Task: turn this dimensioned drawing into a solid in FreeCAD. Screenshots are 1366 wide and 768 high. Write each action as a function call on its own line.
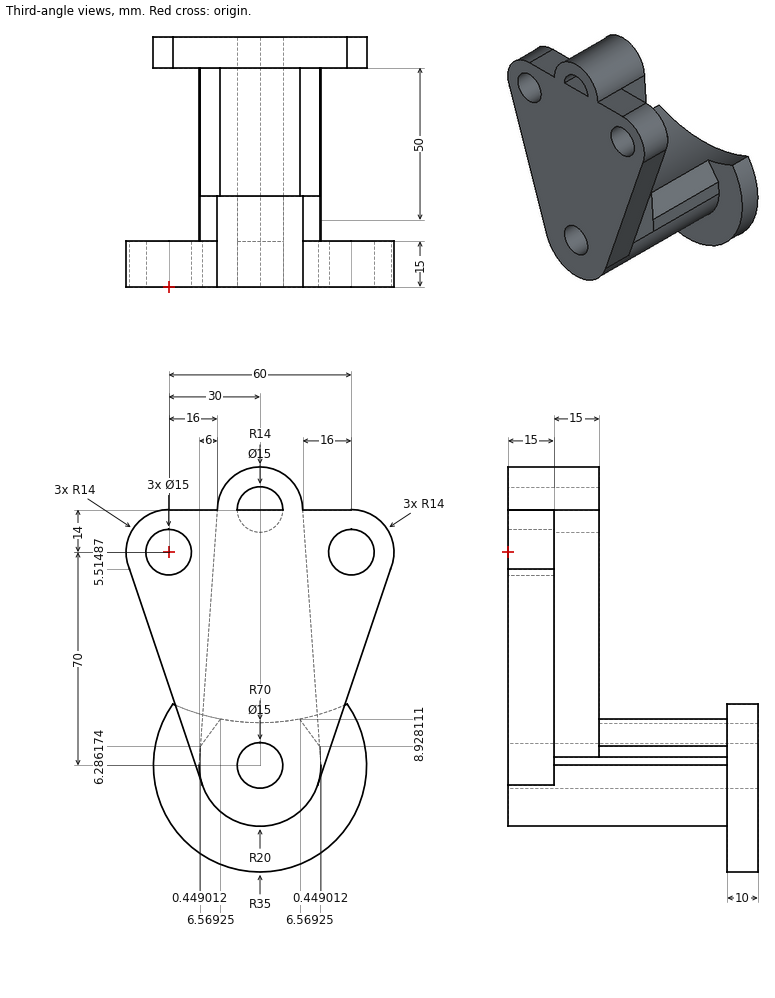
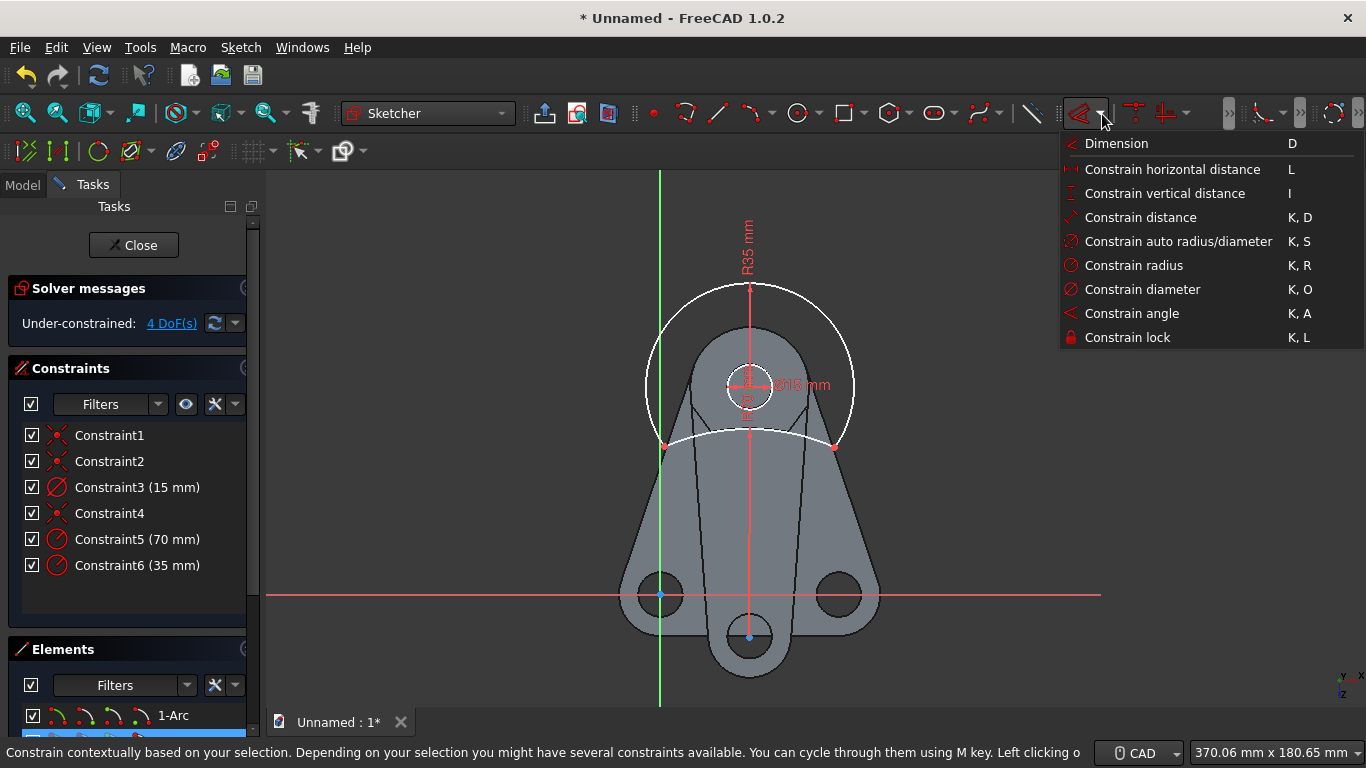
click(1212, 169)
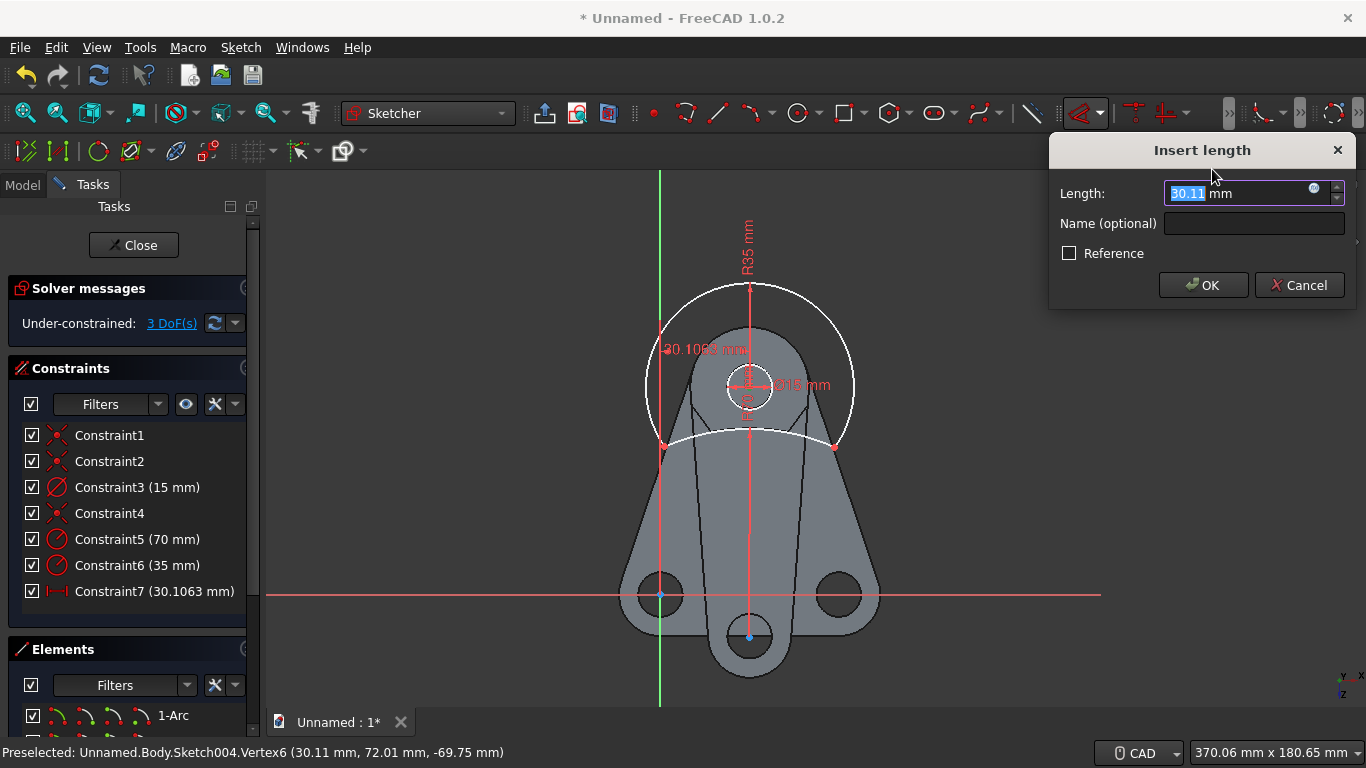
text(30)
key(Return)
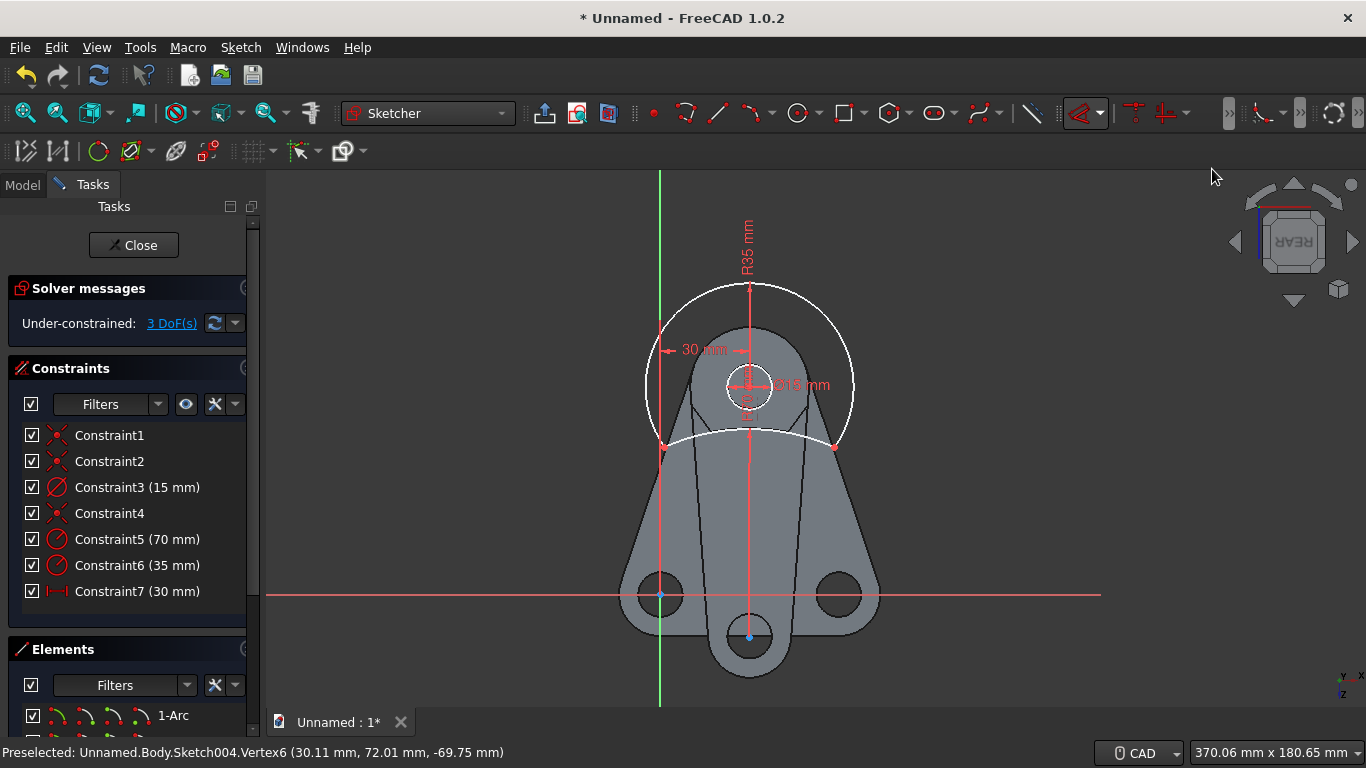
click(750, 387)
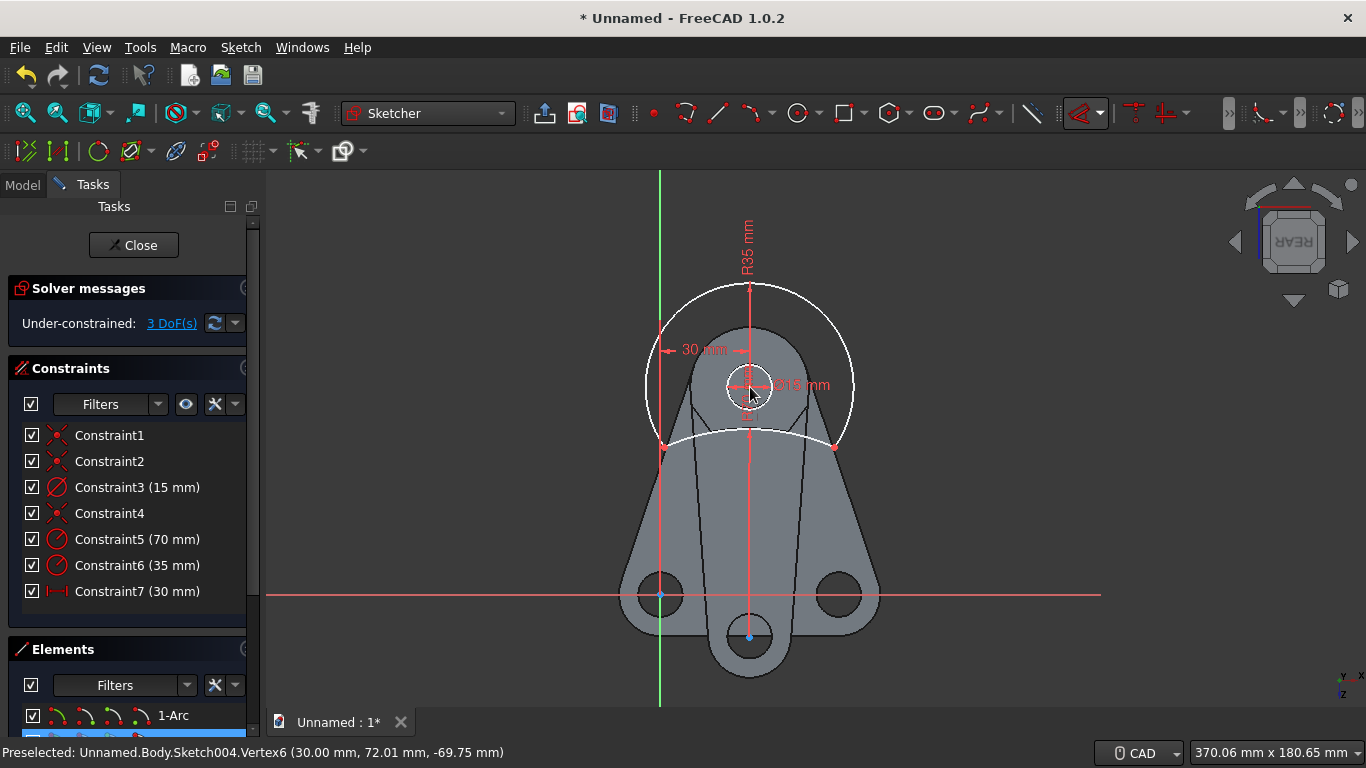
key(i)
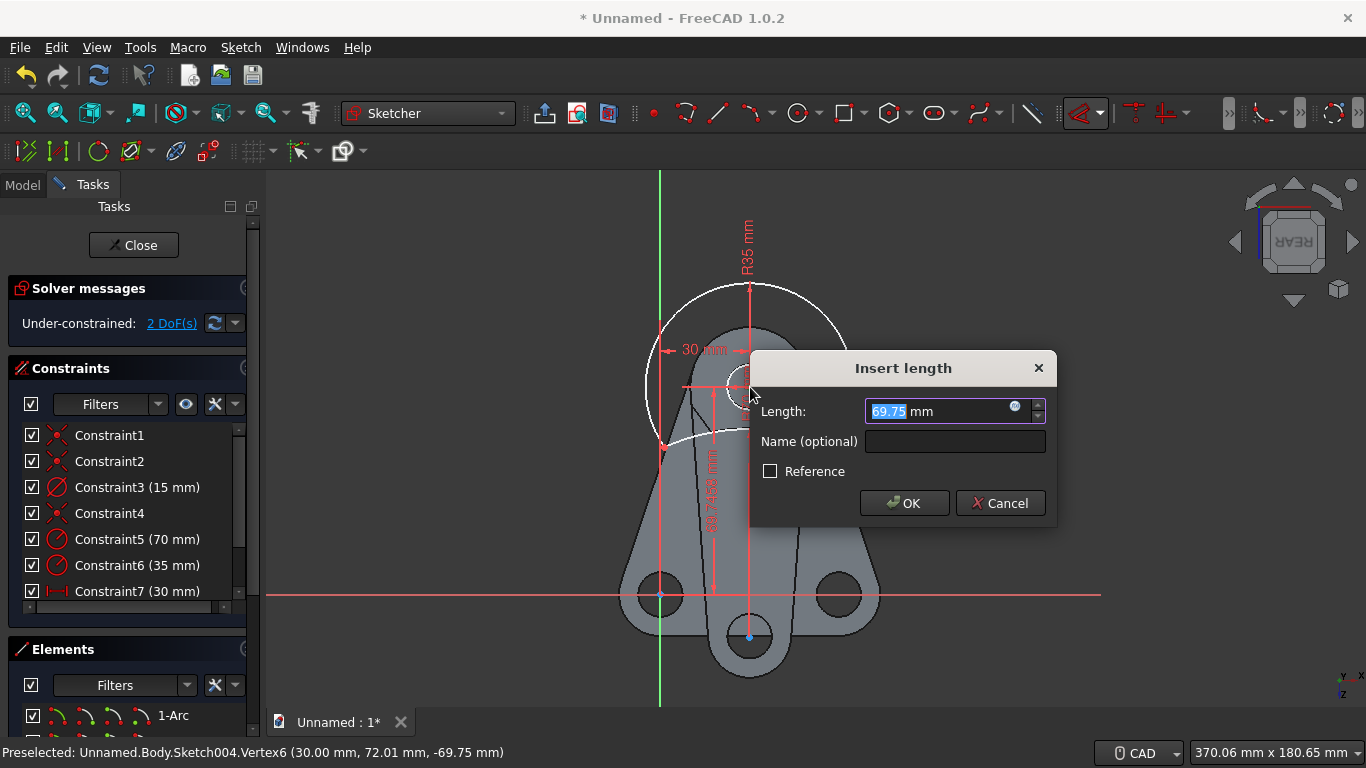
text(70)
key(Return)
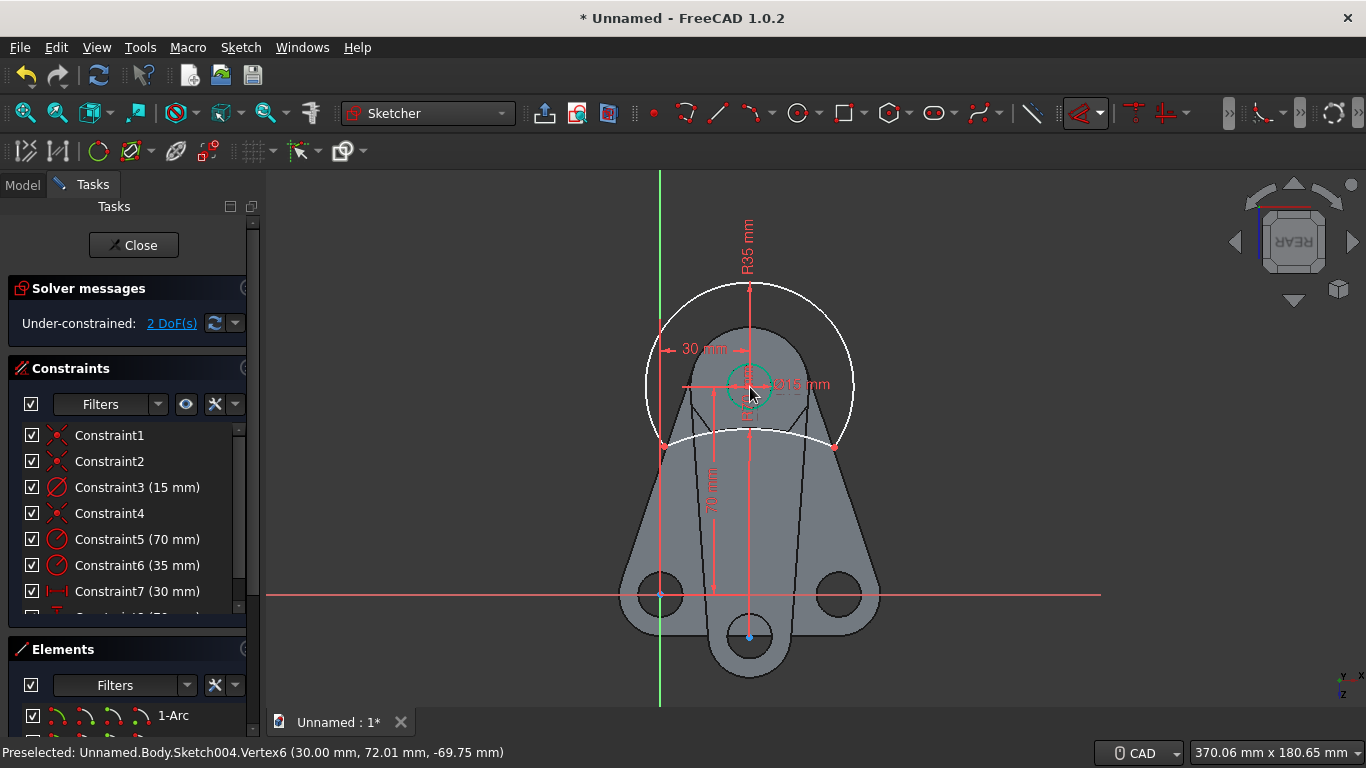
click(749, 637)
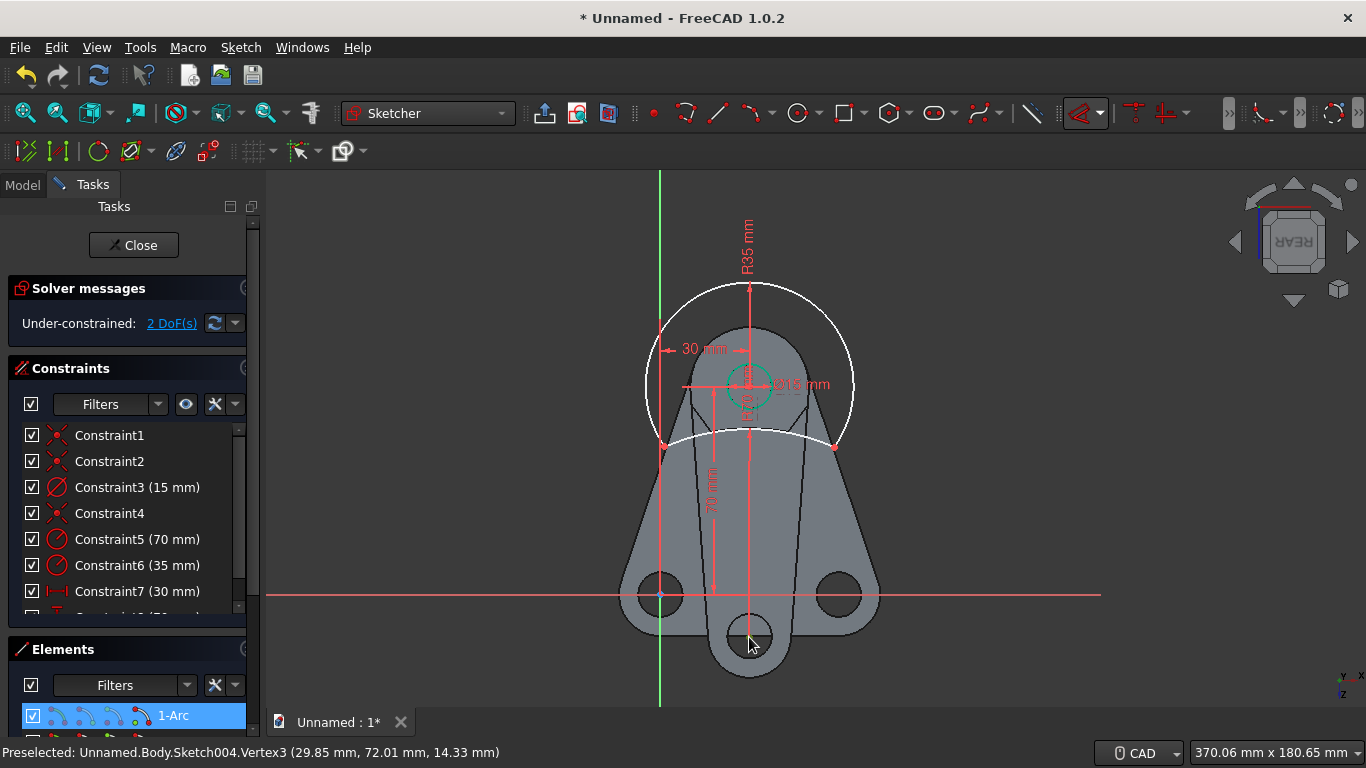
click(1102, 114)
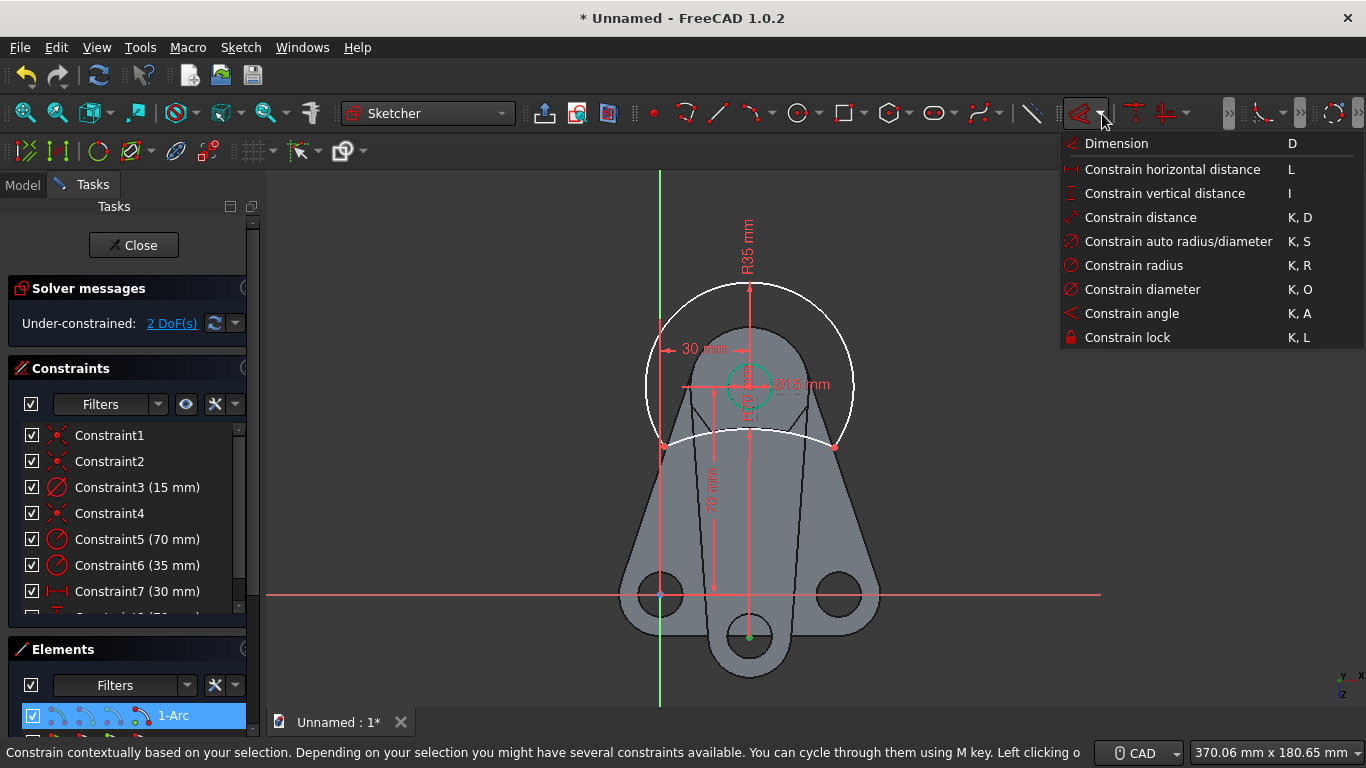
click(1212, 169)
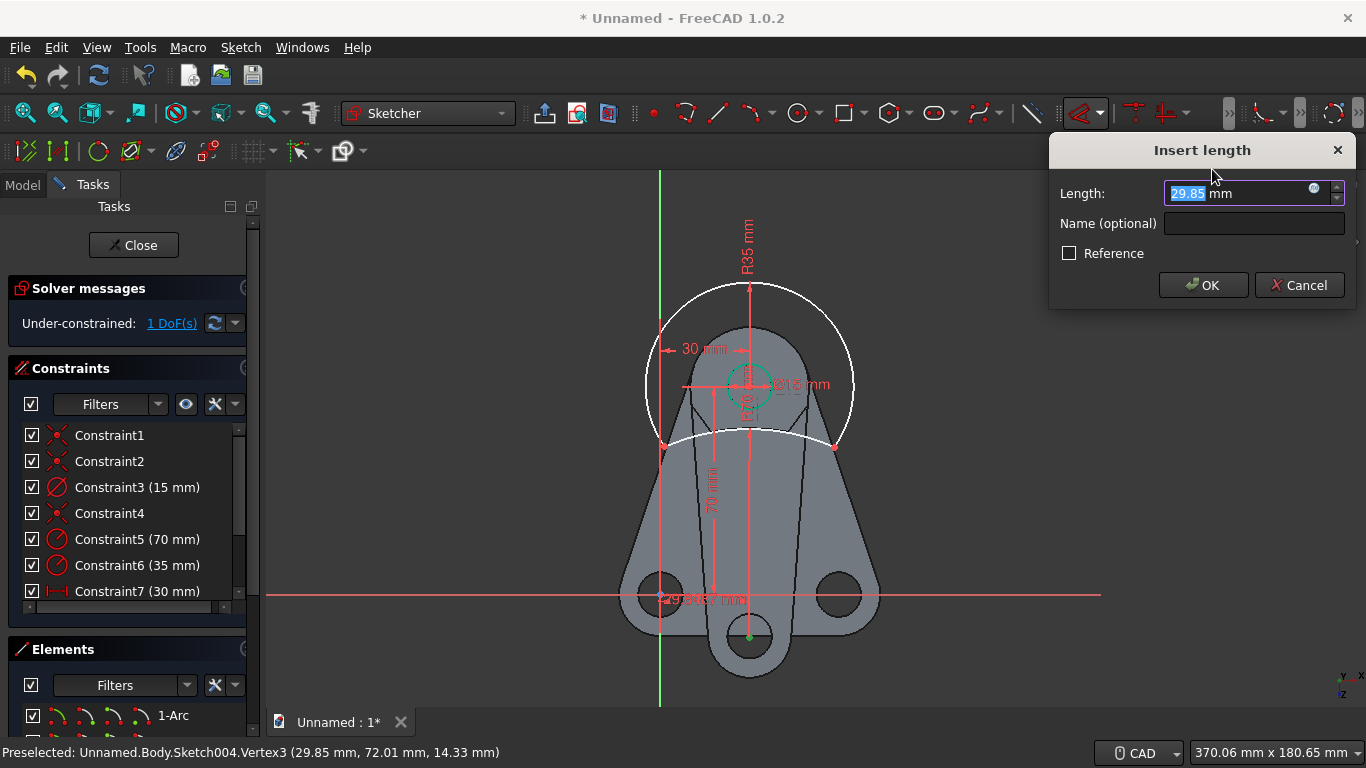
text(30)
key(Return)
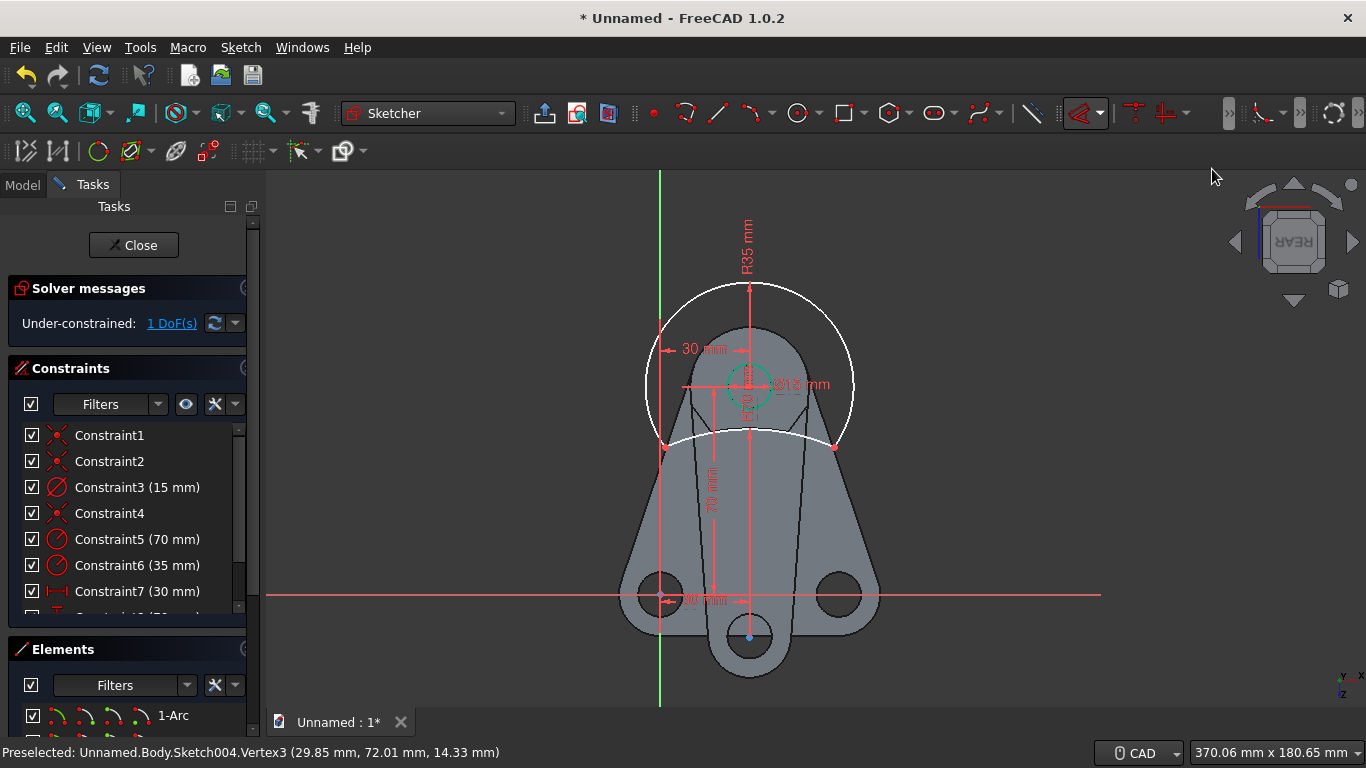
click(750, 637)